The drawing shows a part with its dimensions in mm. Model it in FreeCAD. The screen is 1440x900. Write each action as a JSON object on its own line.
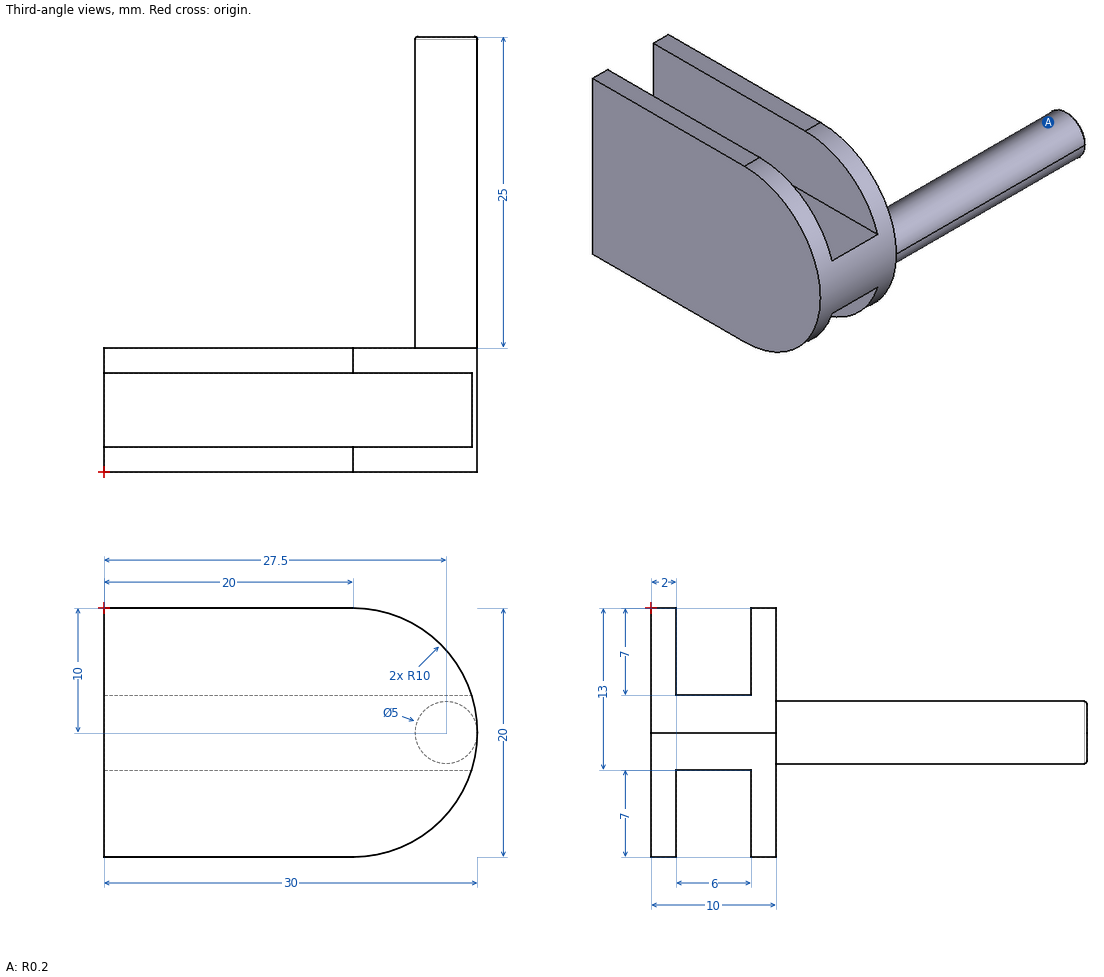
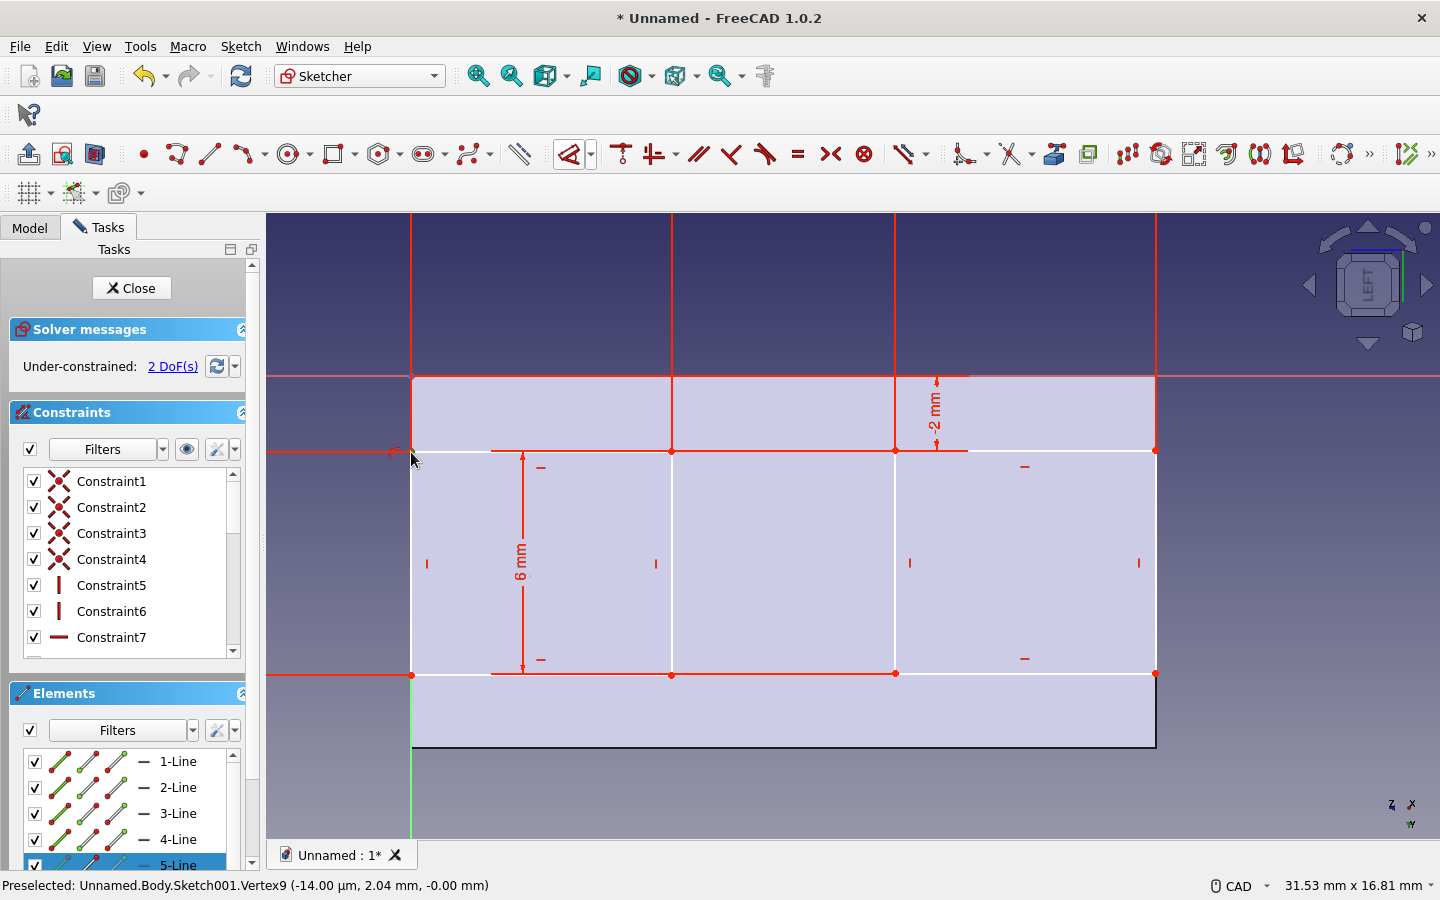
{"action": "left_click", "coordinate": [590, 154]}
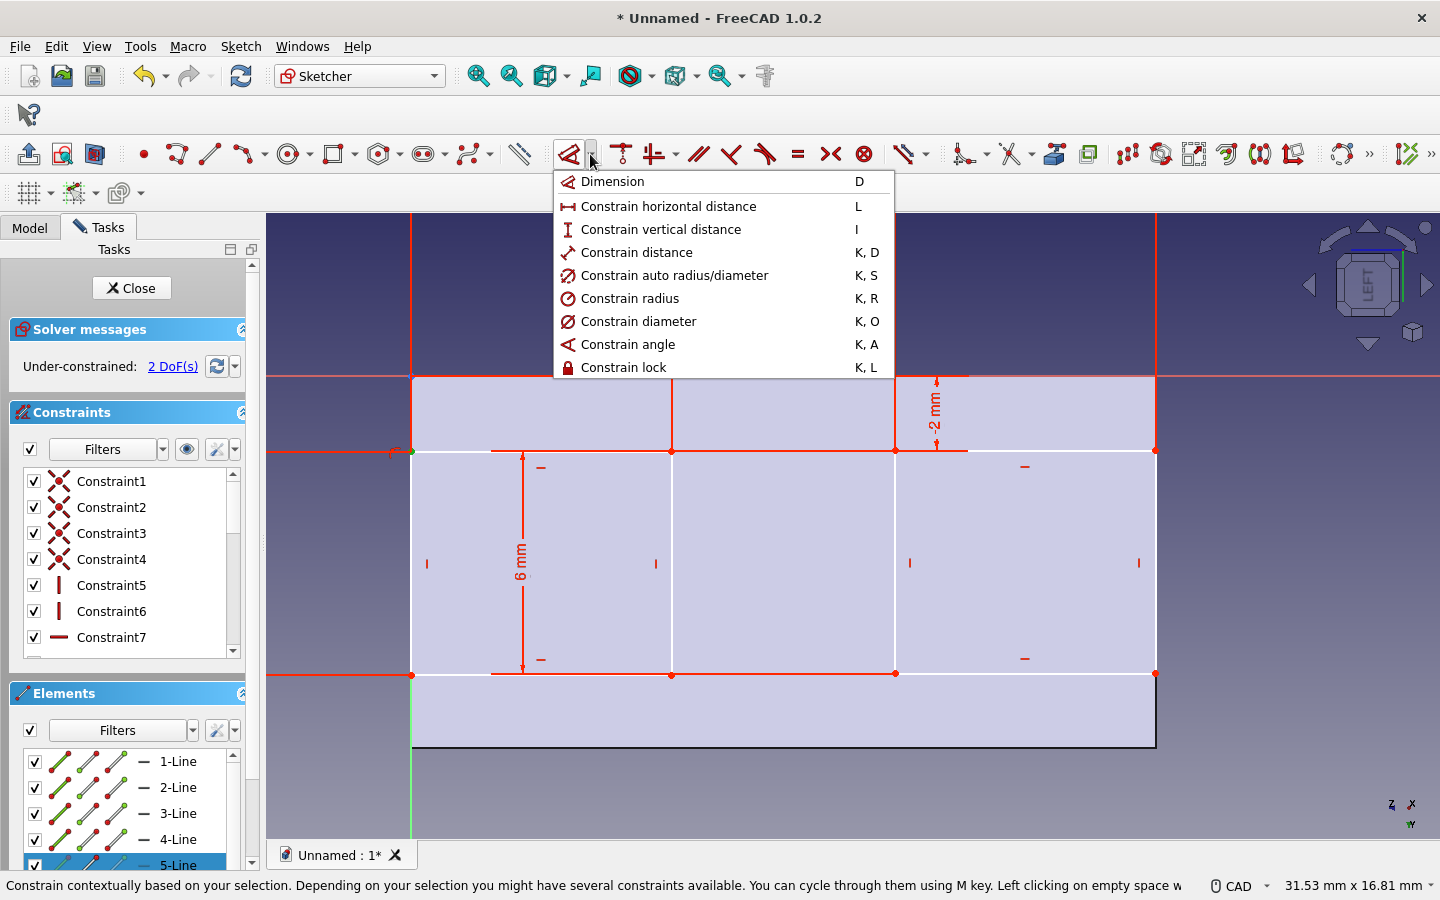
{"action": "left_click", "coordinate": [724, 230]}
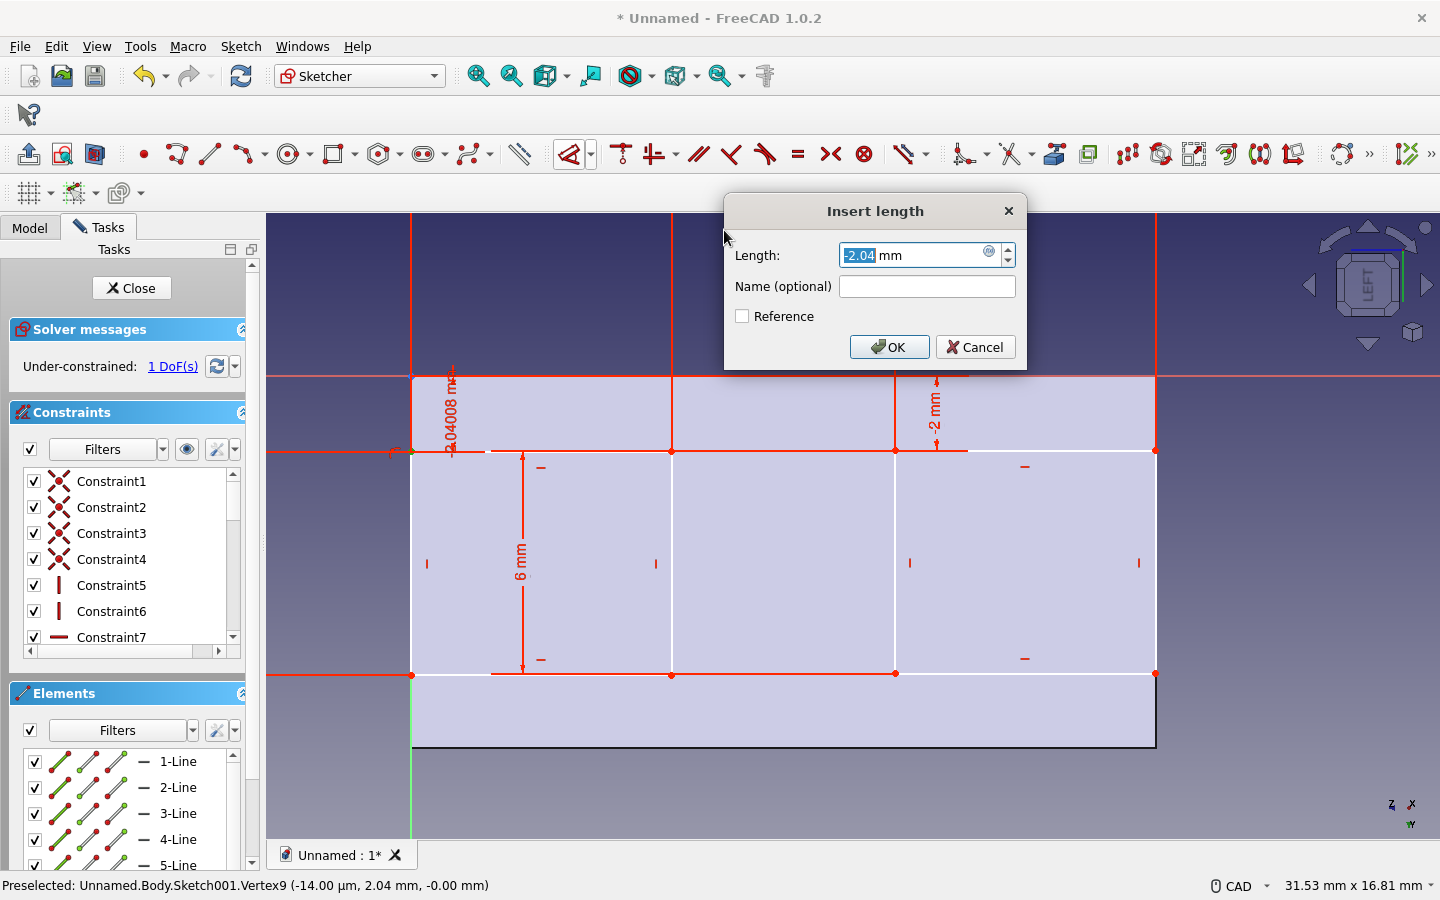
{"action": "type", "text": "-2"}
{"action": "key", "text": "Return"}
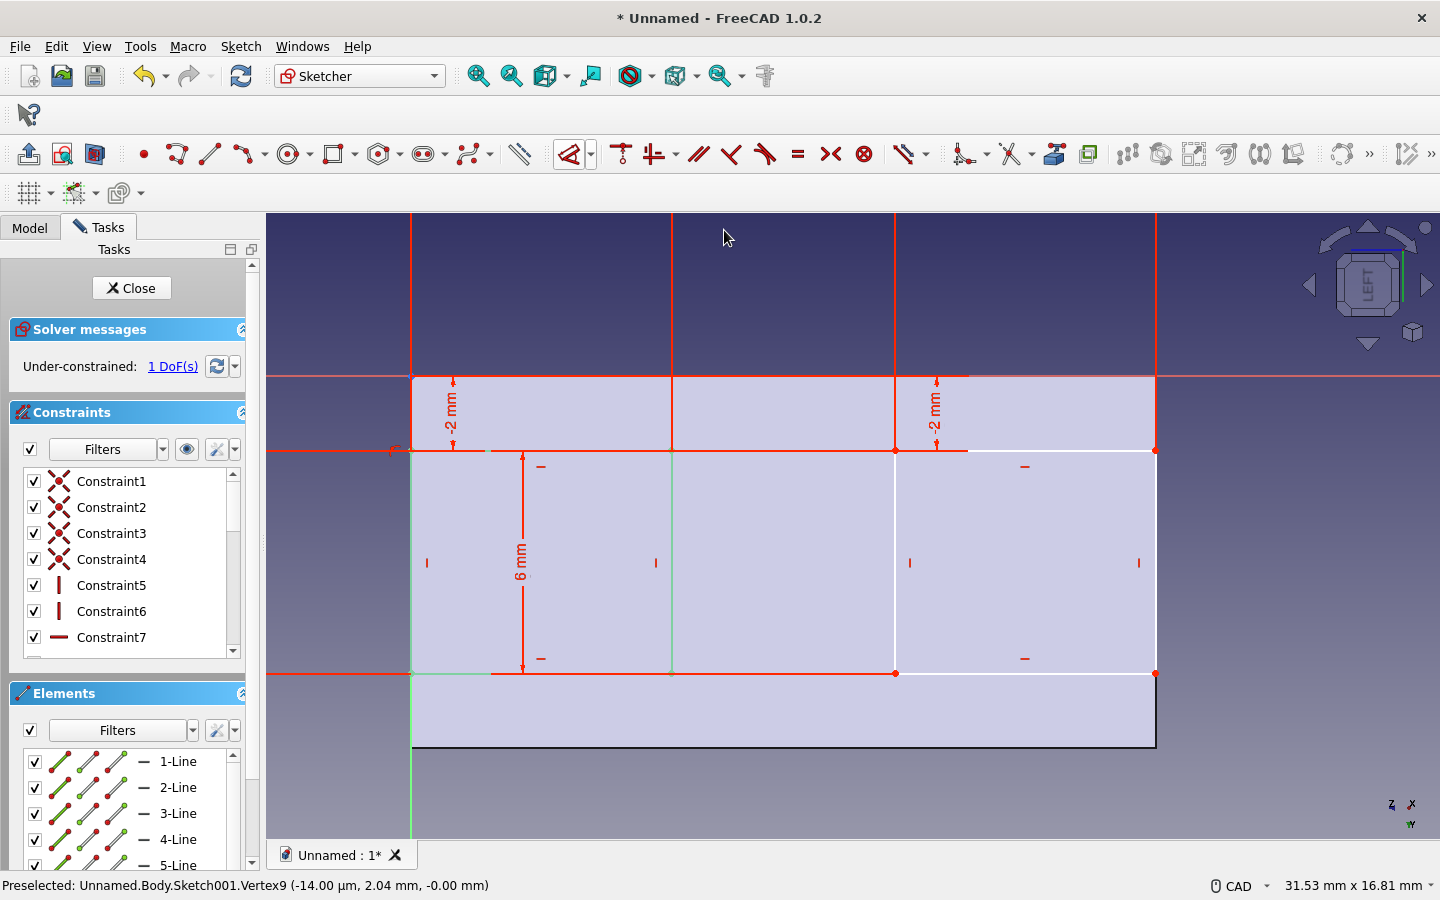
{"action": "left_click", "coordinate": [895, 451]}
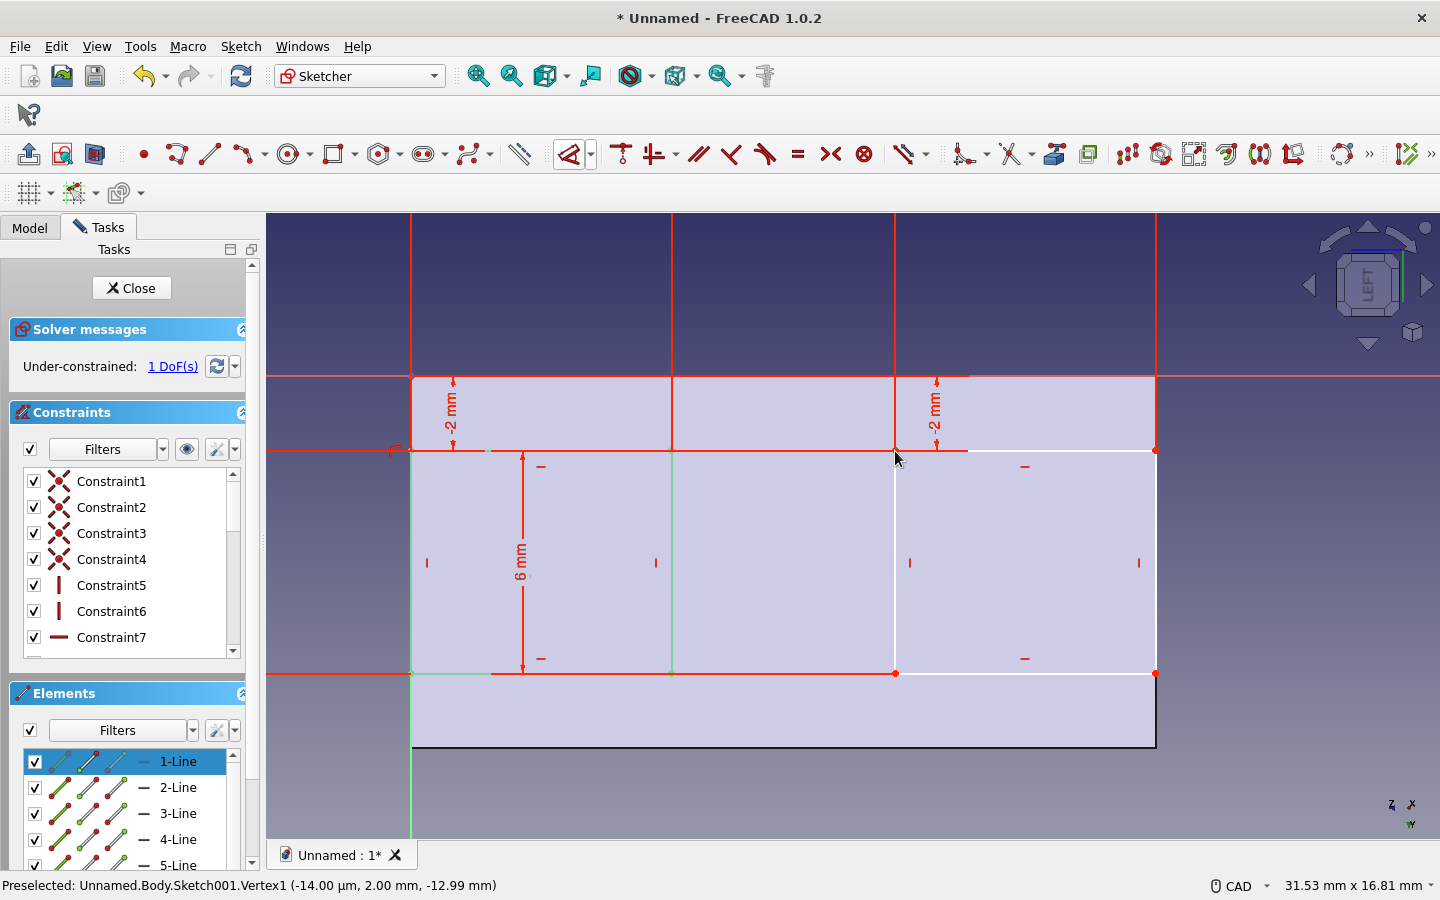
{"action": "left_click", "coordinate": [590, 154]}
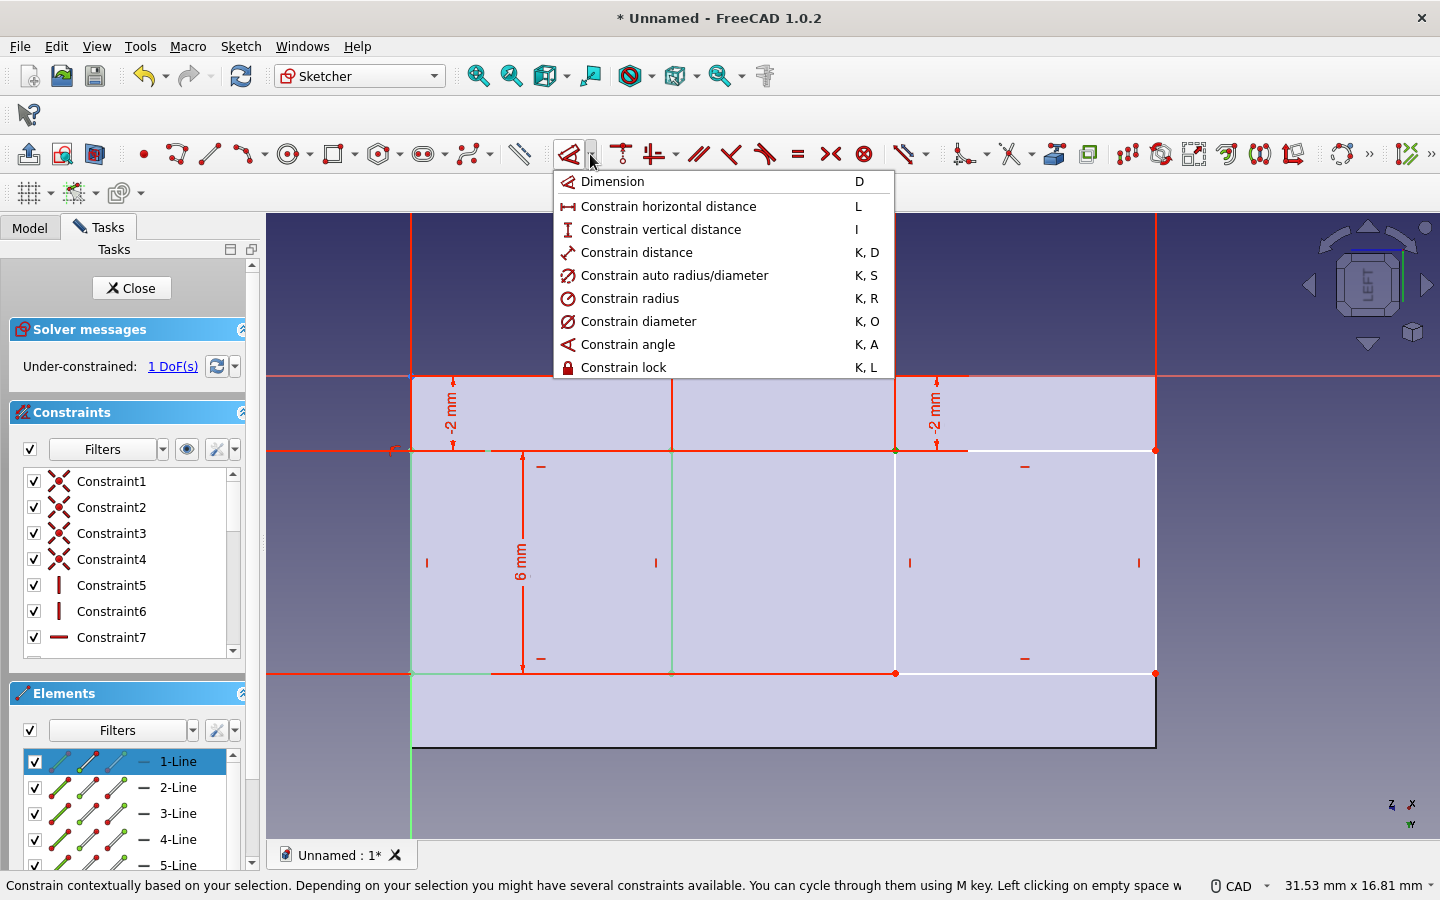
{"action": "left_click", "coordinate": [724, 206]}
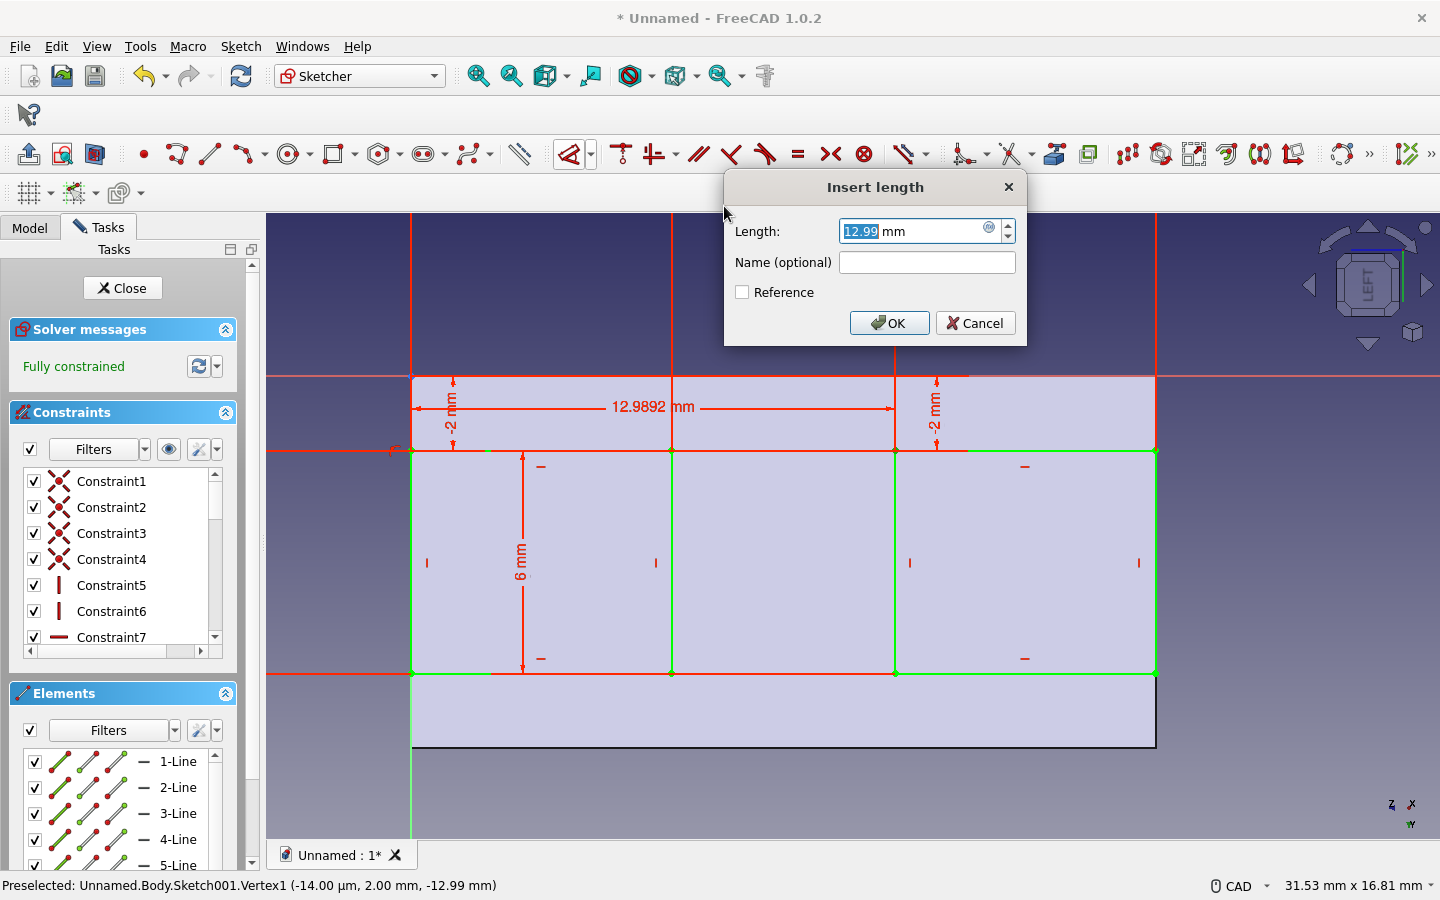
{"action": "type", "text": "13"}
{"action": "key", "text": "Return"}